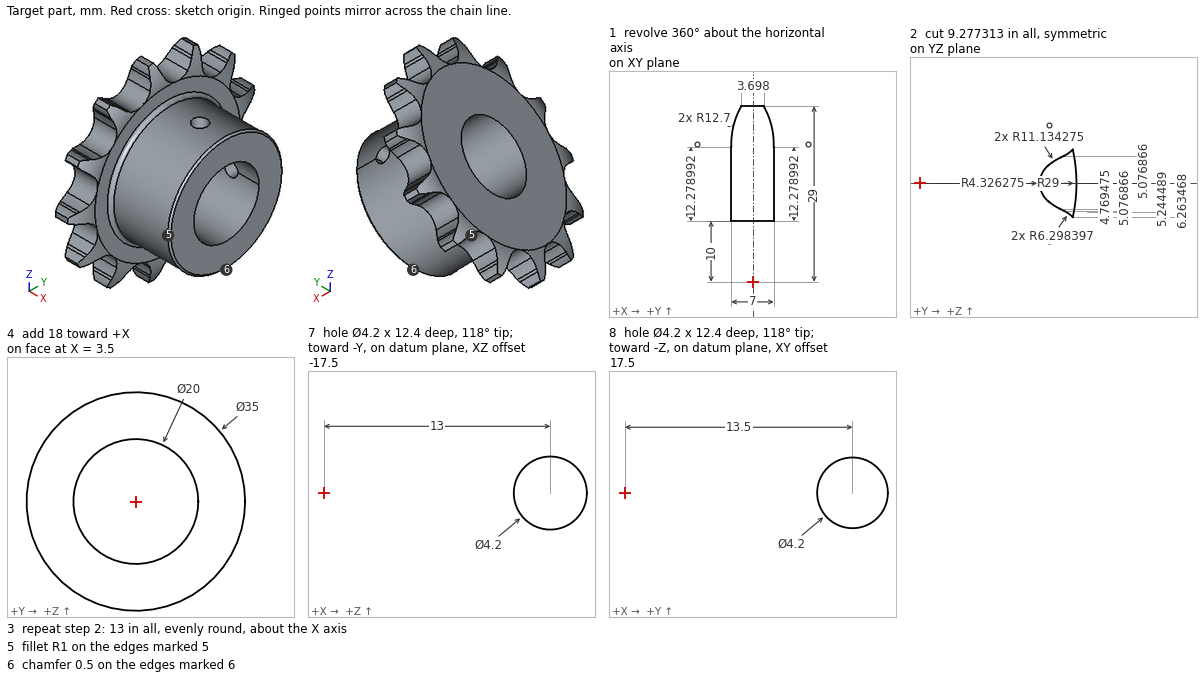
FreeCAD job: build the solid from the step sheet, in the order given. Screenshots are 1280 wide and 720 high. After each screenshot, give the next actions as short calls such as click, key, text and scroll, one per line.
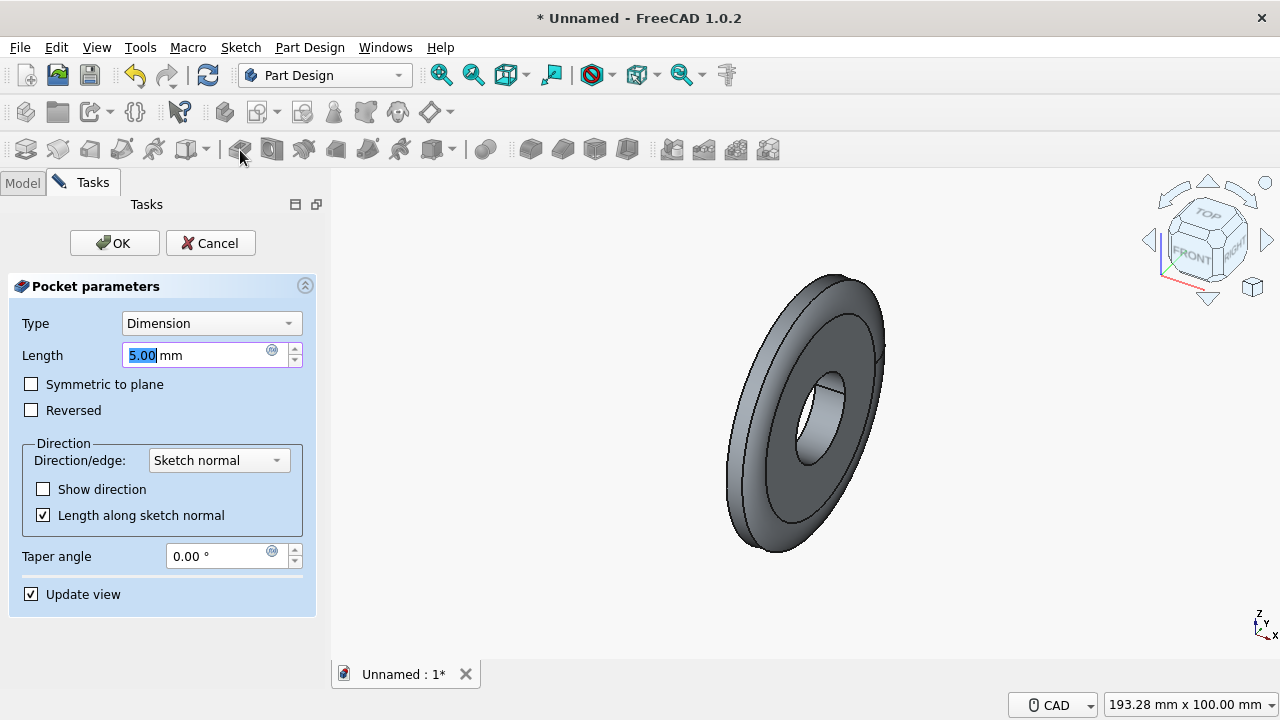
text(9.277313)
key(Tab)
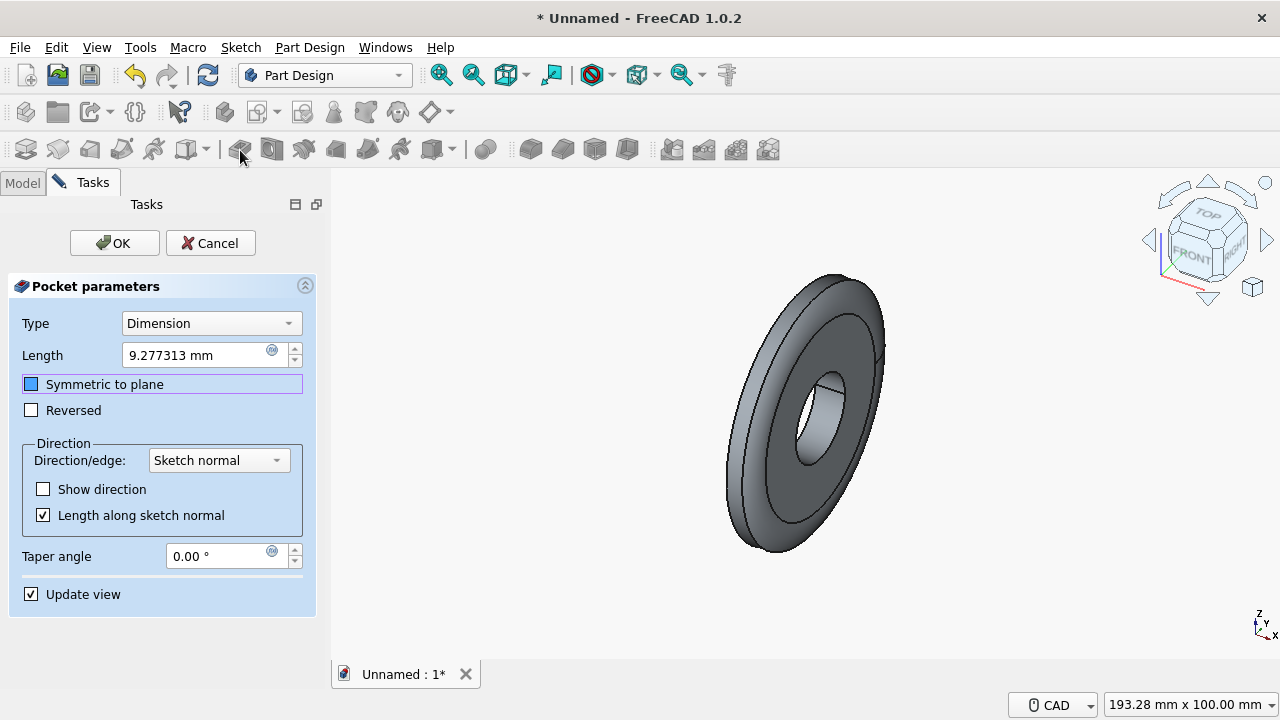
click(30, 384)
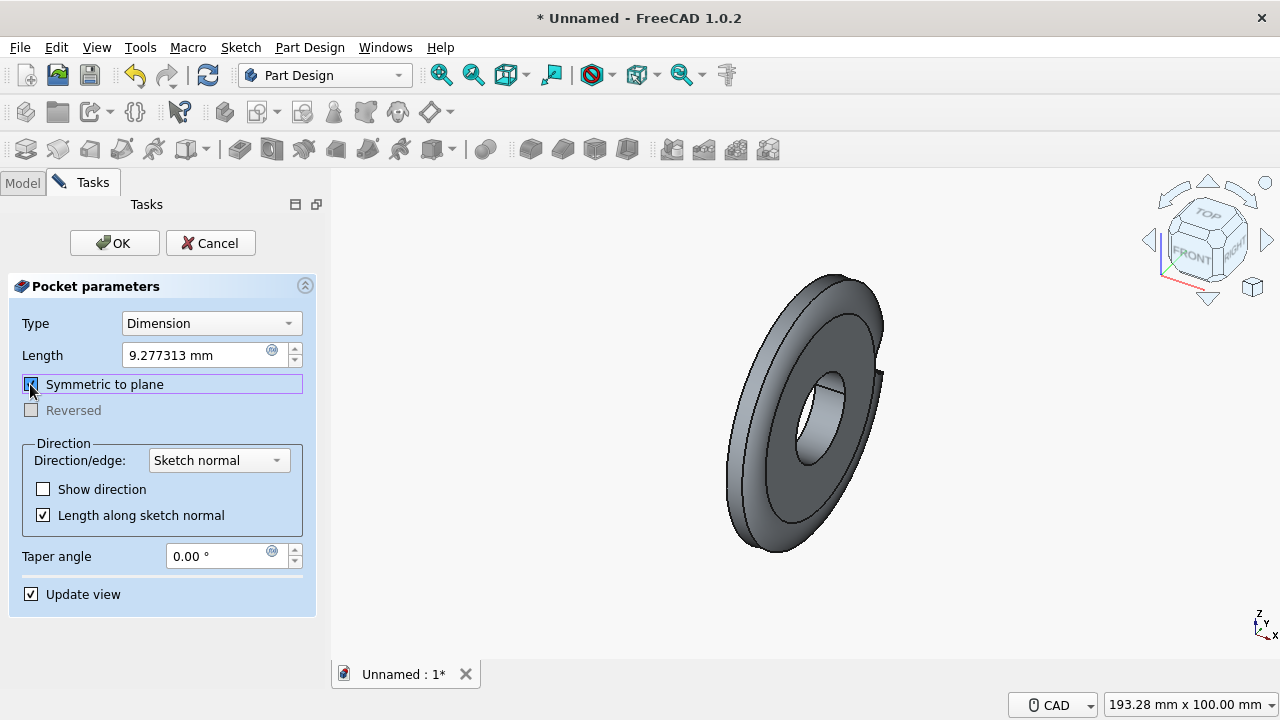
click(115, 243)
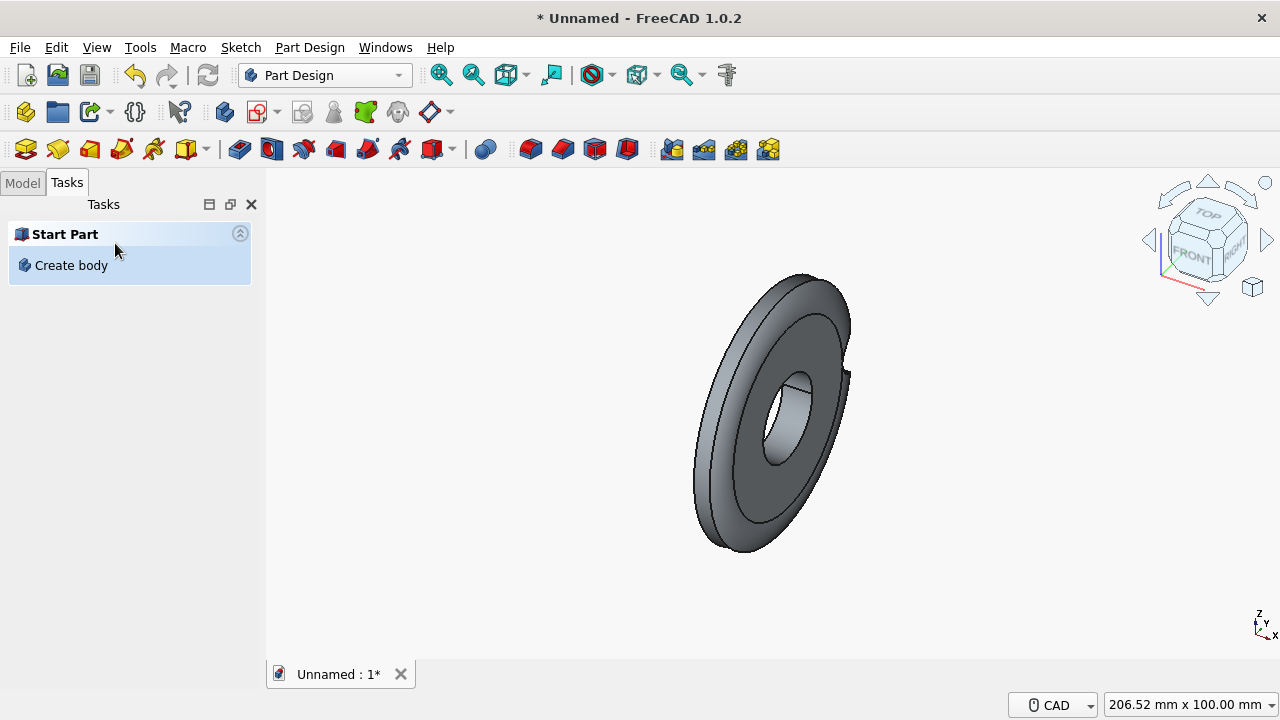
click(23, 182)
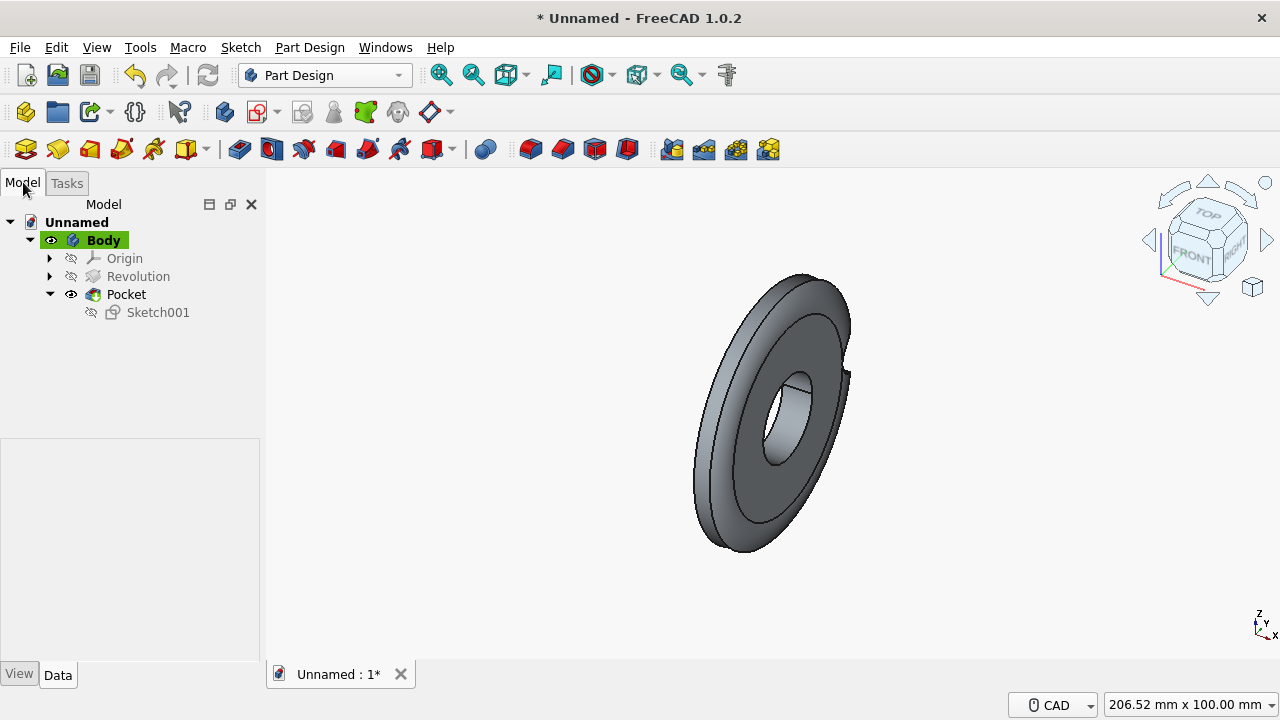
click(116, 294)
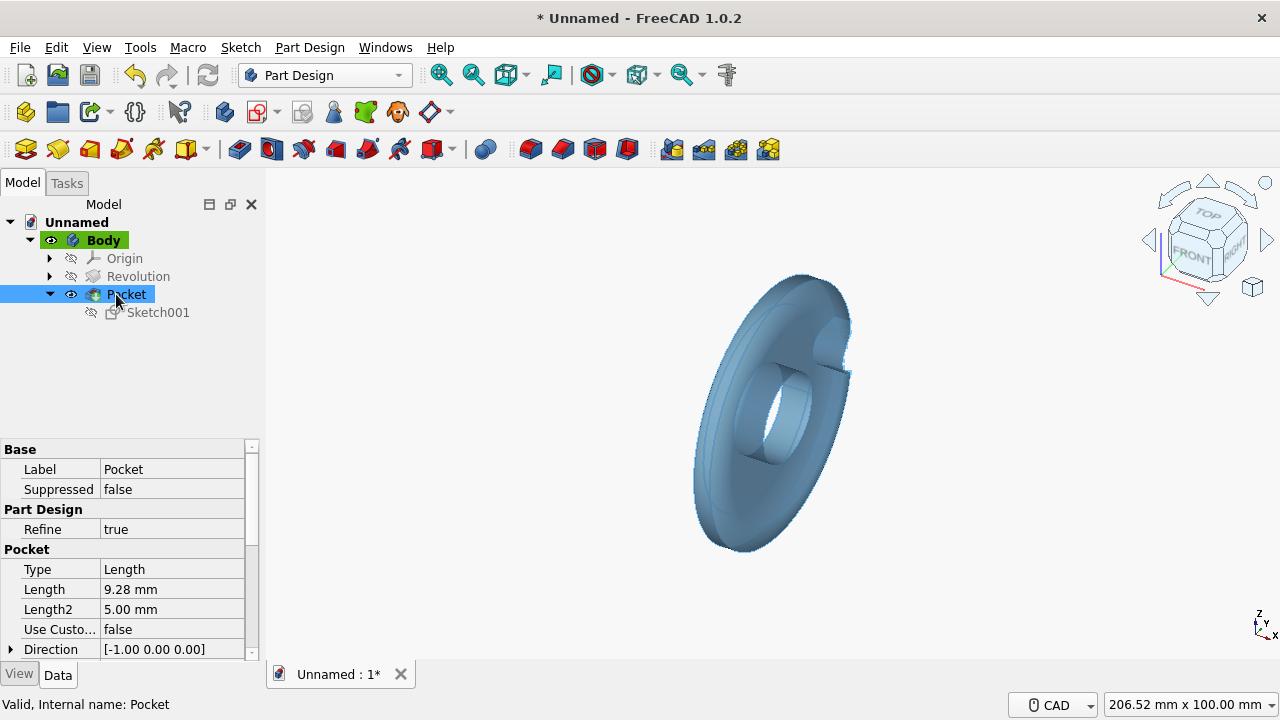
click(736, 150)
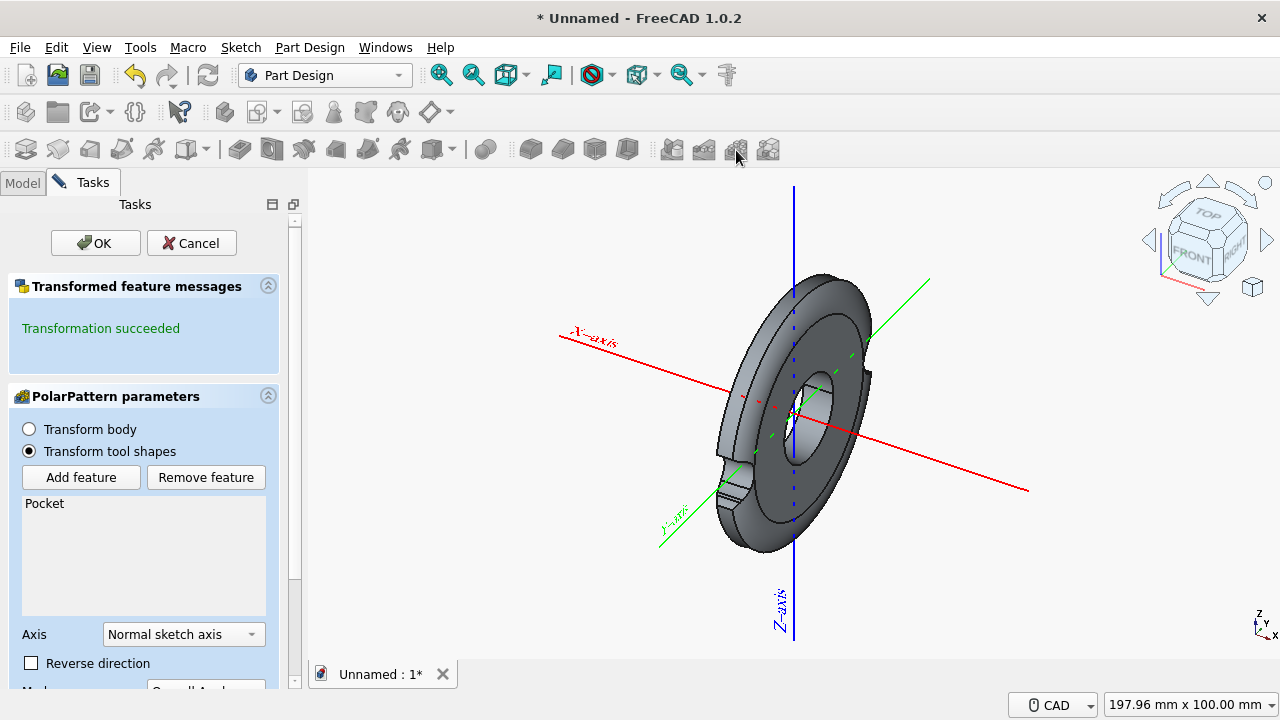
click(184, 634)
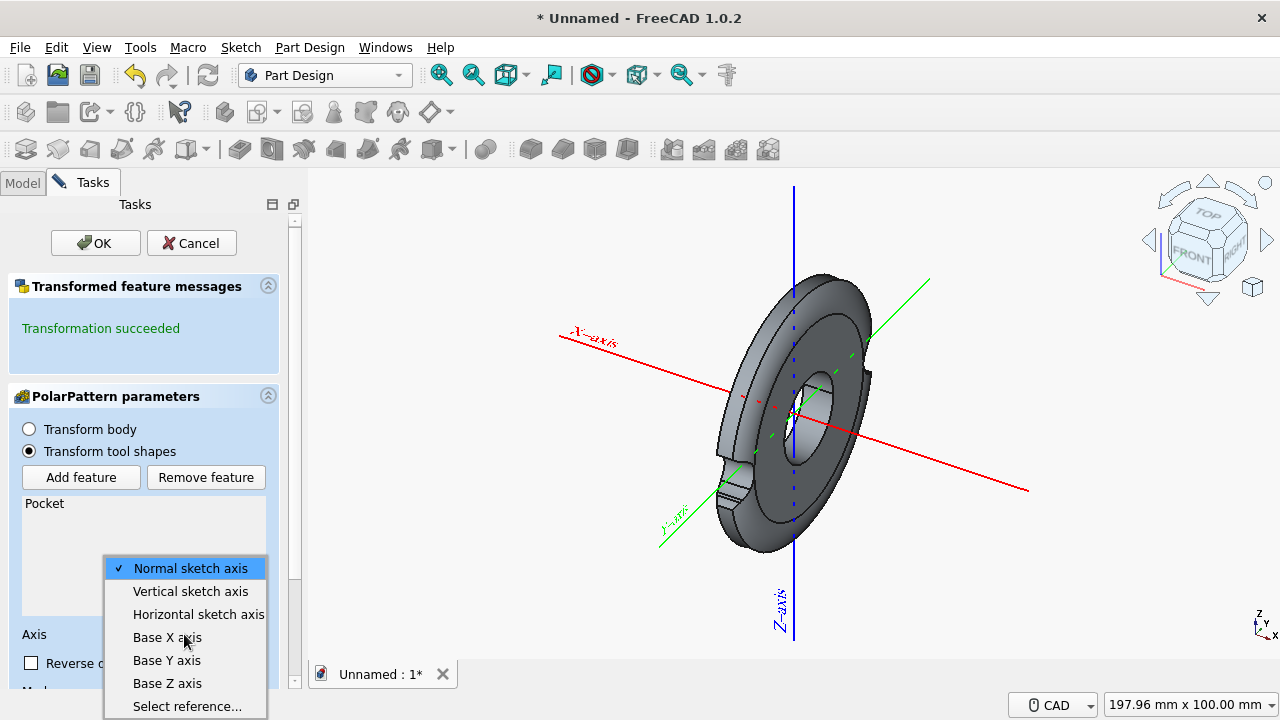
click(184, 638)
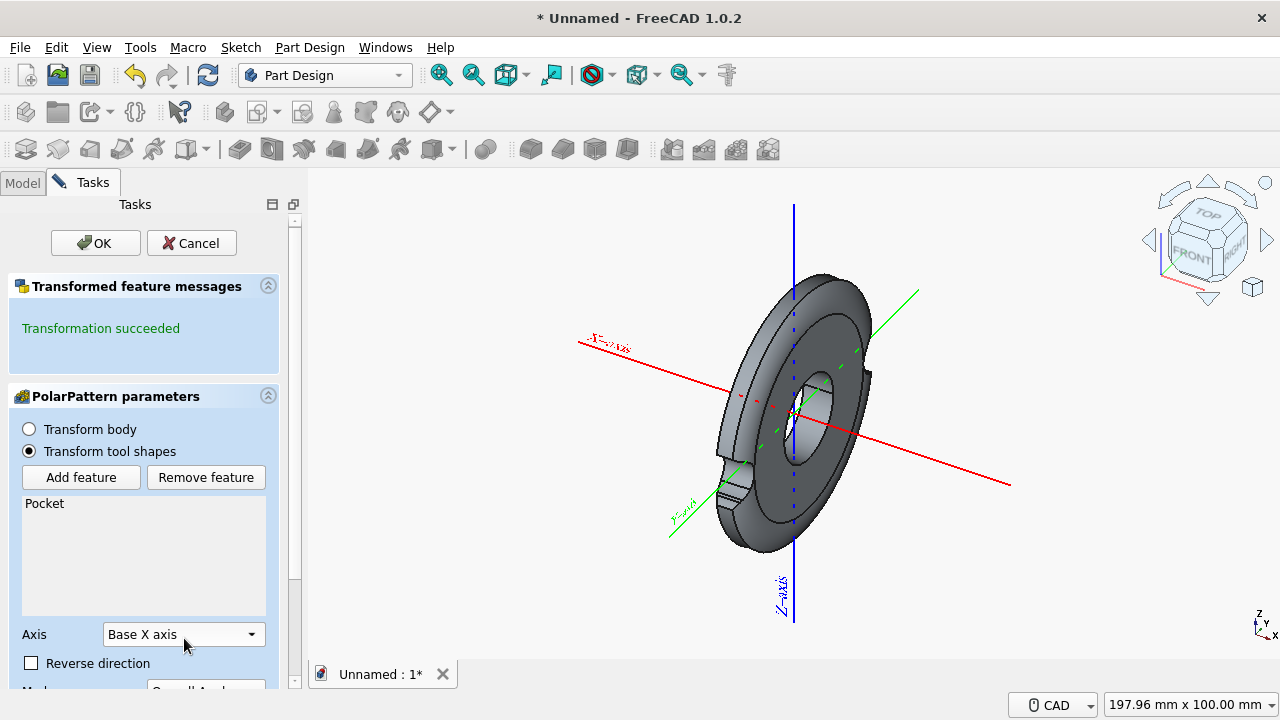
scroll(295, 451, down, 3)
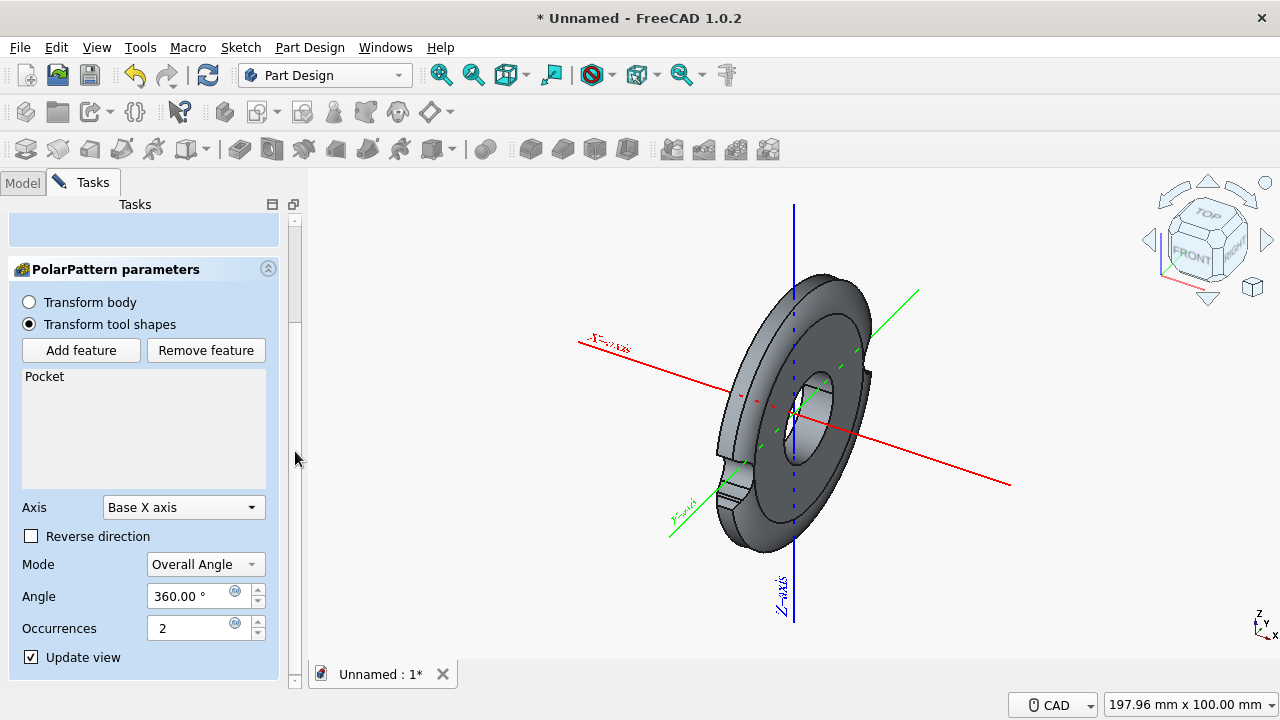
triple_click(198, 628)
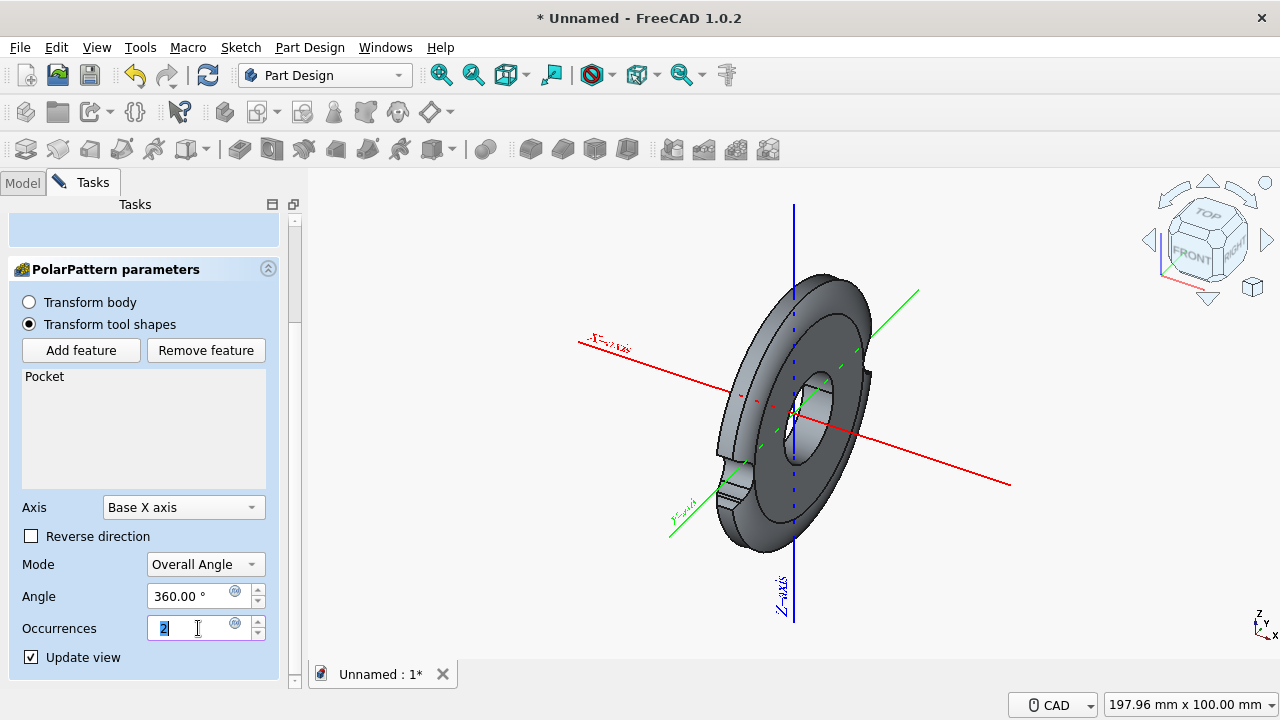
text(13)
key(Tab)